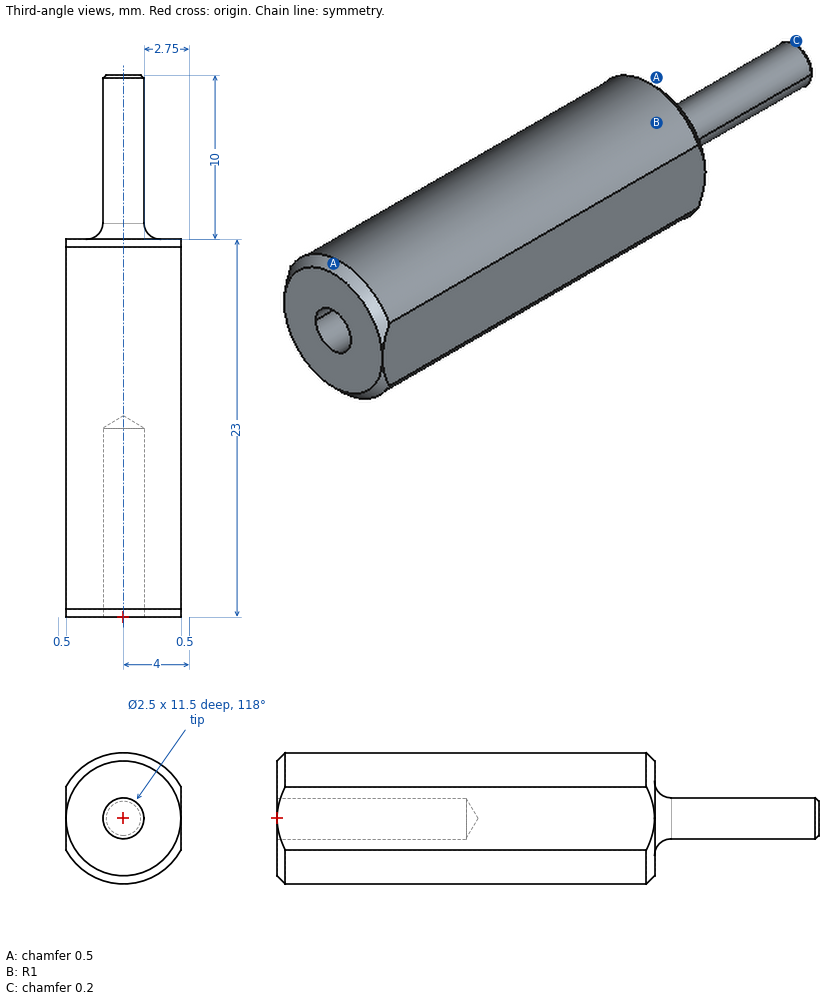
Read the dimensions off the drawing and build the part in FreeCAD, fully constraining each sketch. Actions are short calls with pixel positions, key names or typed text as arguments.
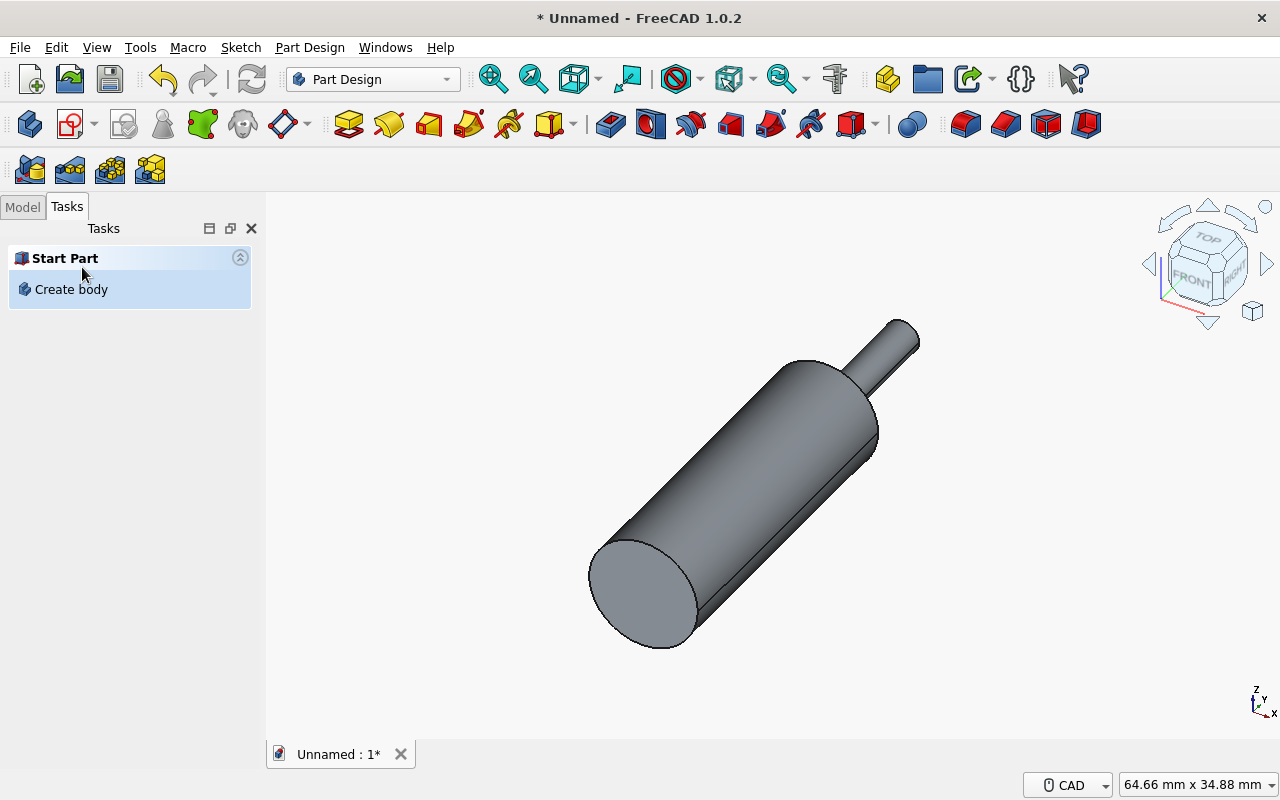
click(70, 124)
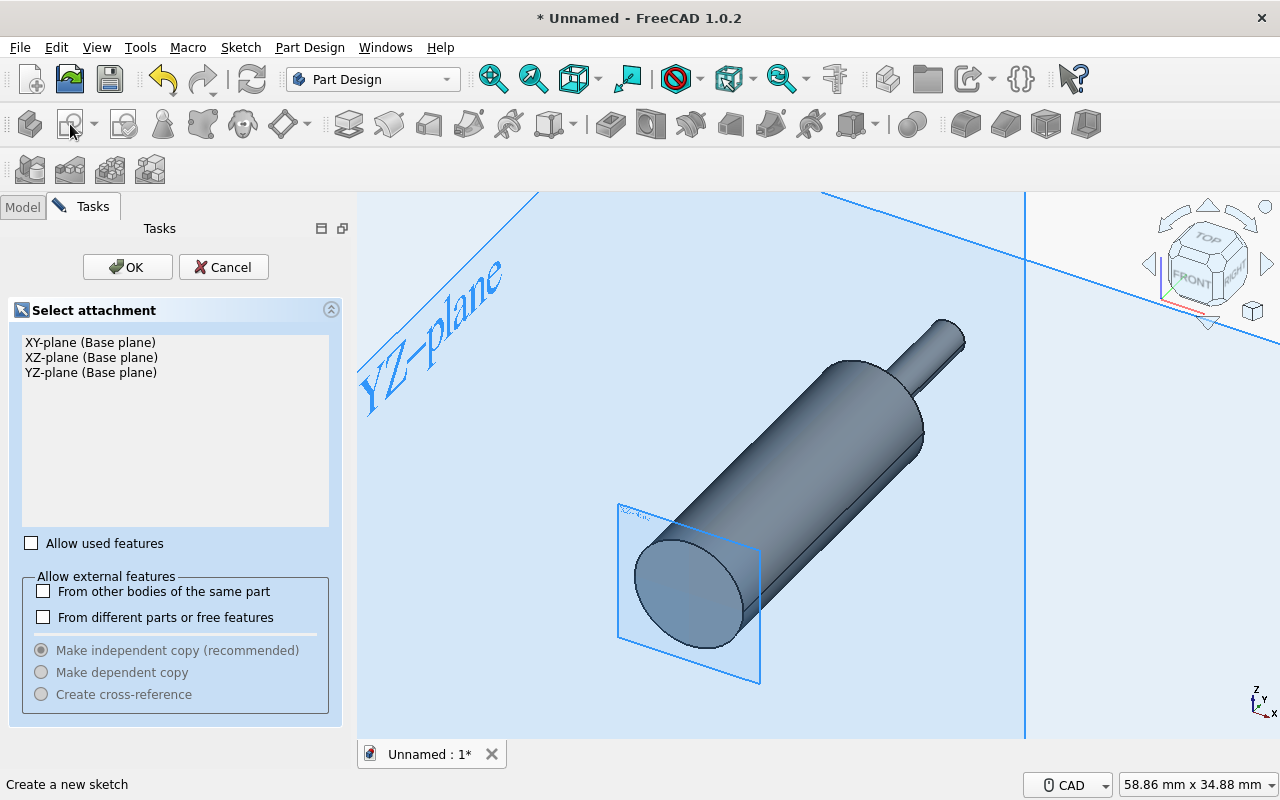
click(82, 358)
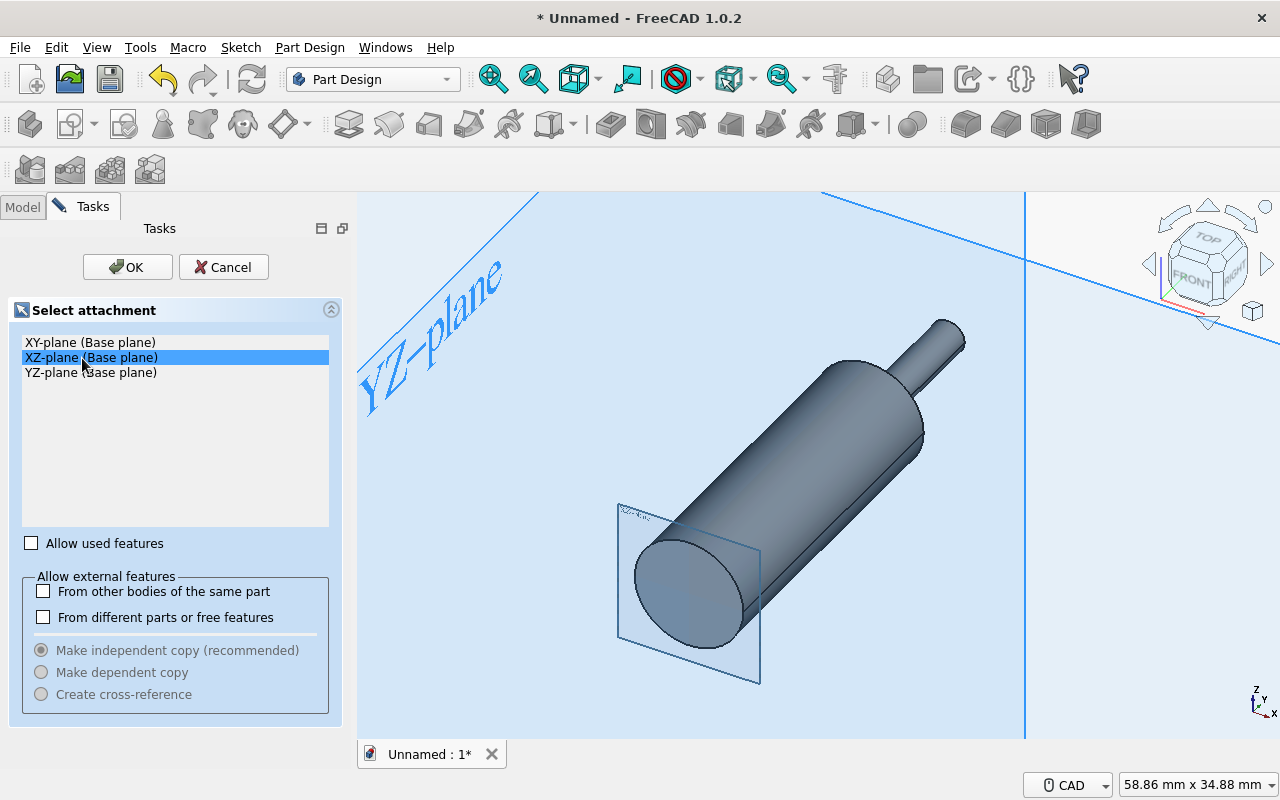
click(128, 267)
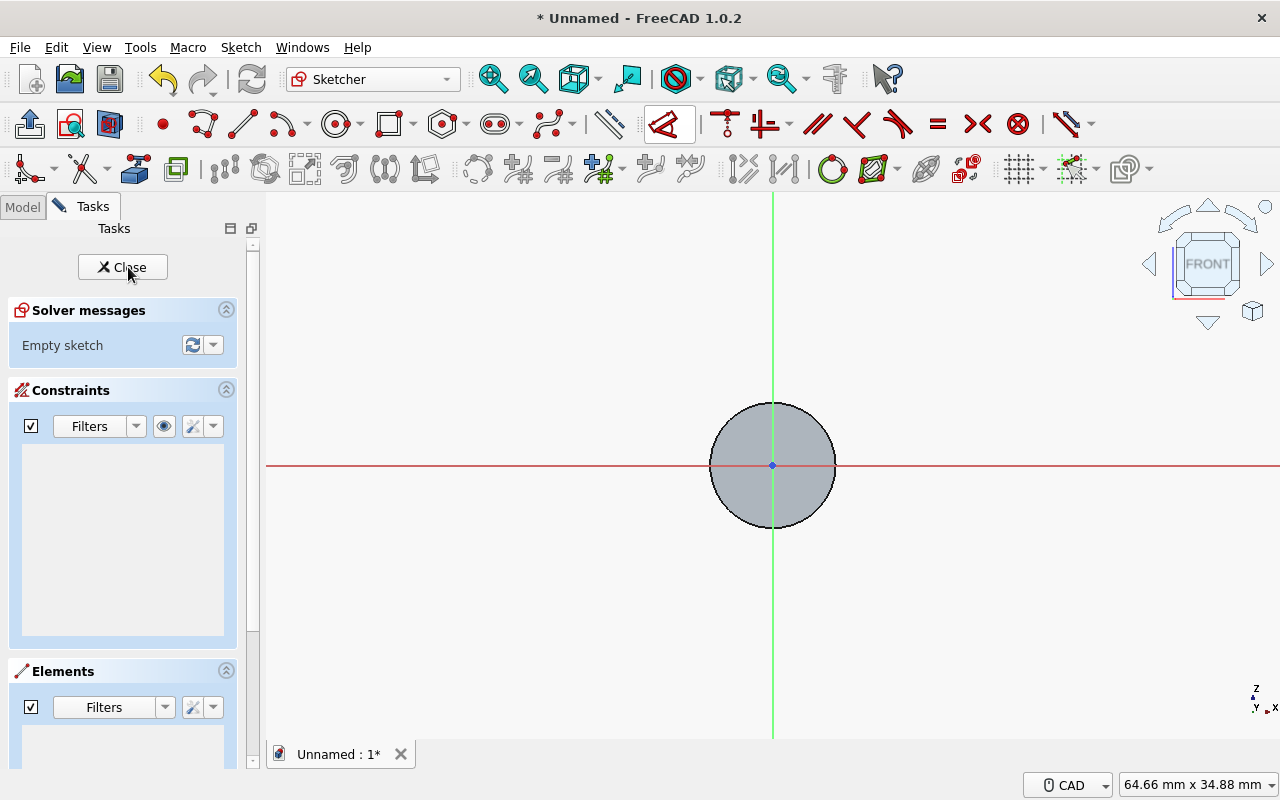
scroll(781, 466, up, 11)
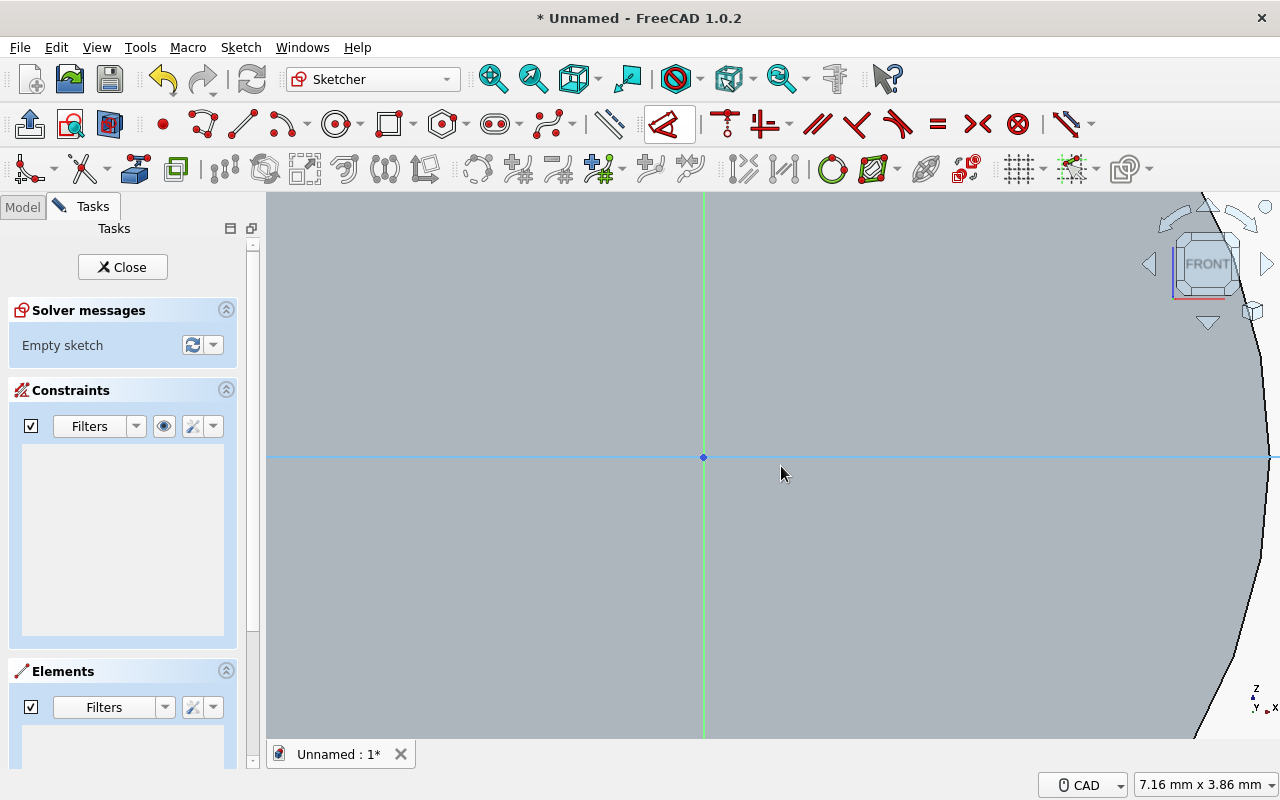
key(g)
key(c)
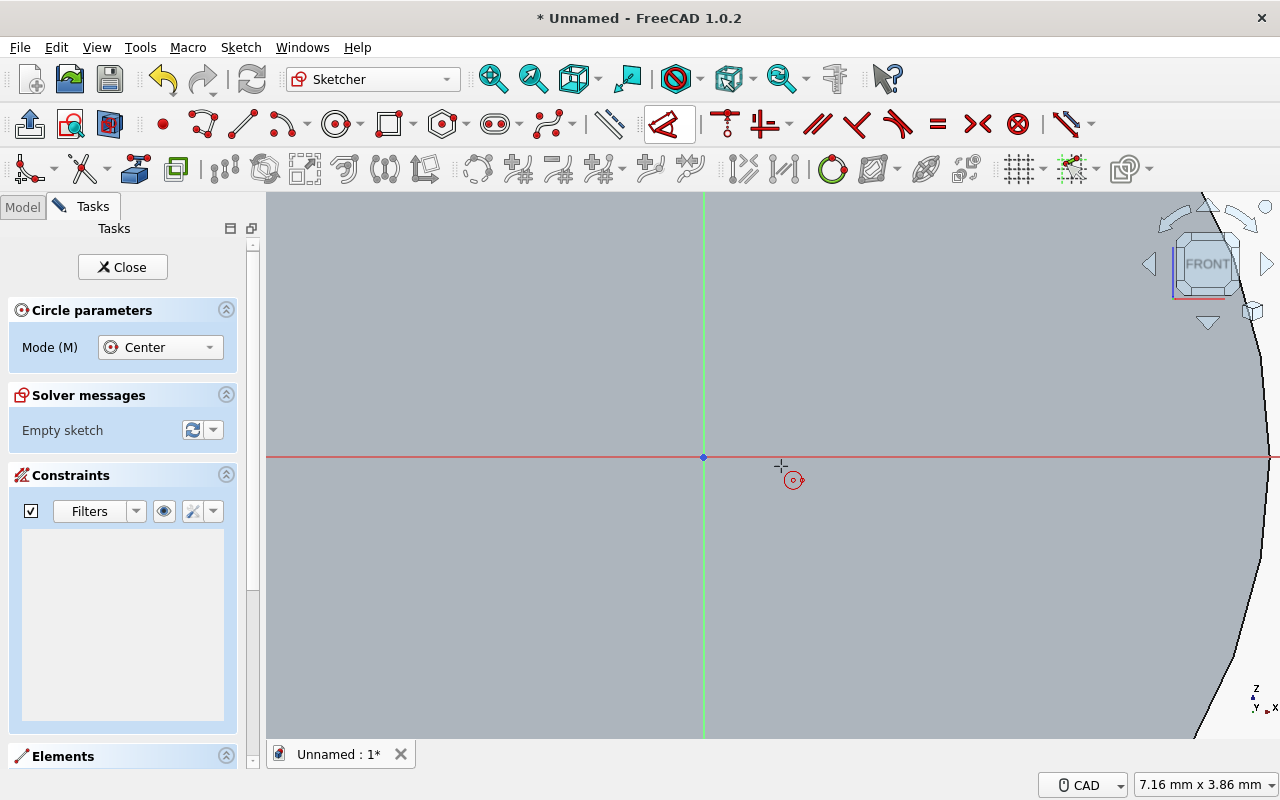
click(704, 457)
move(829, 332)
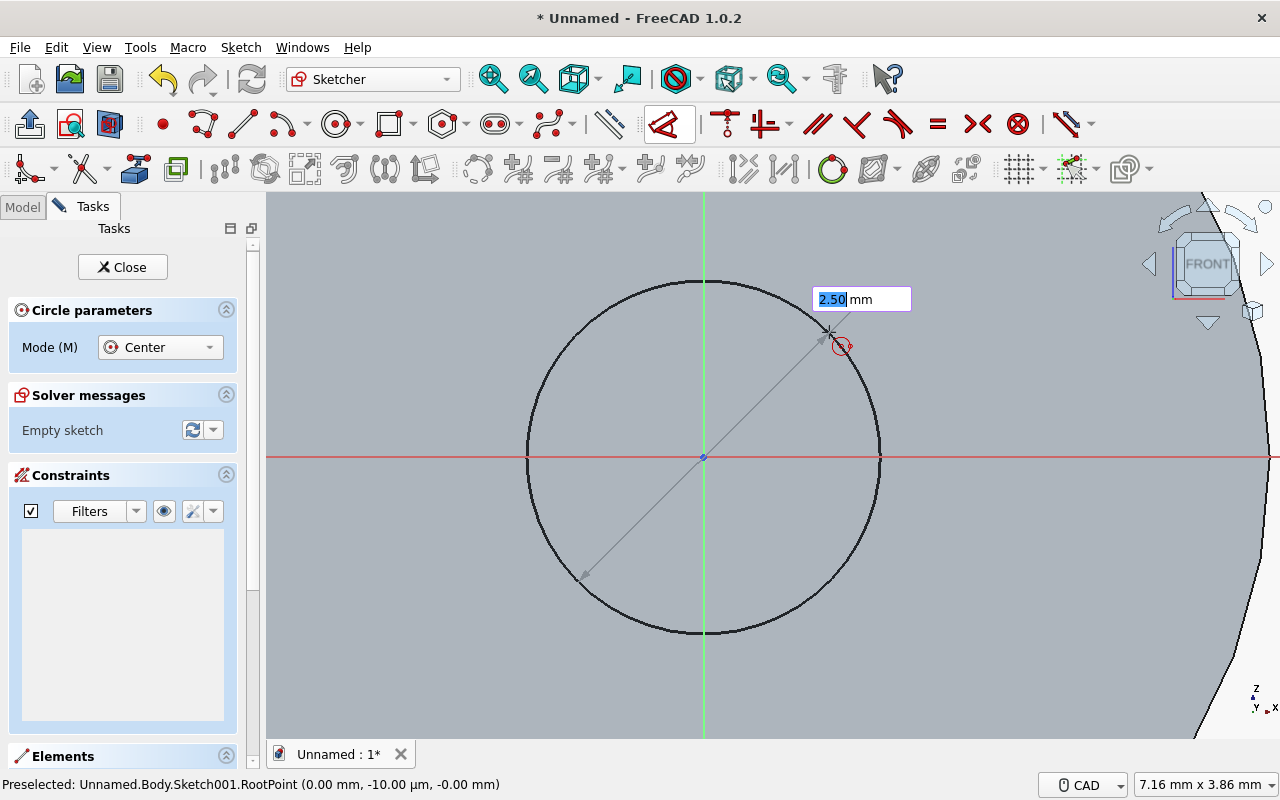
text(2.5)
key(Return)
key(Escape)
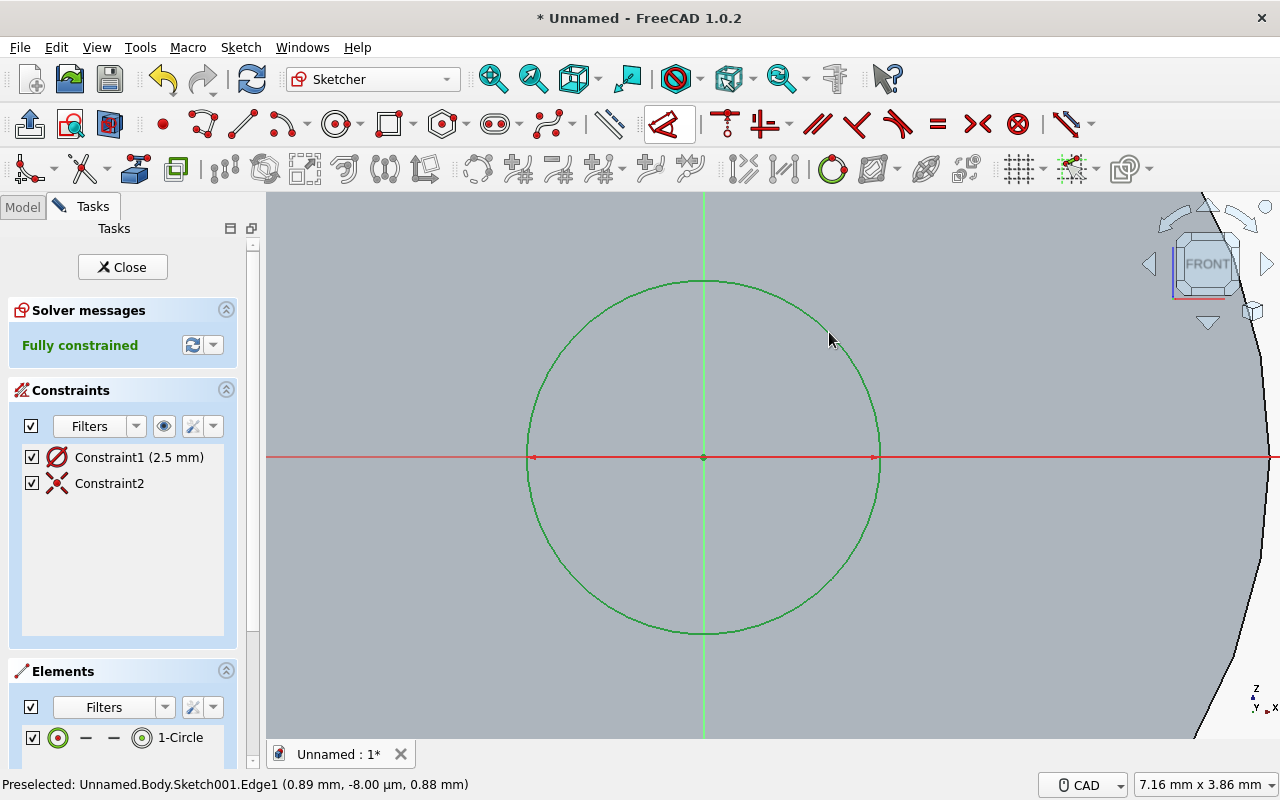
click(123, 267)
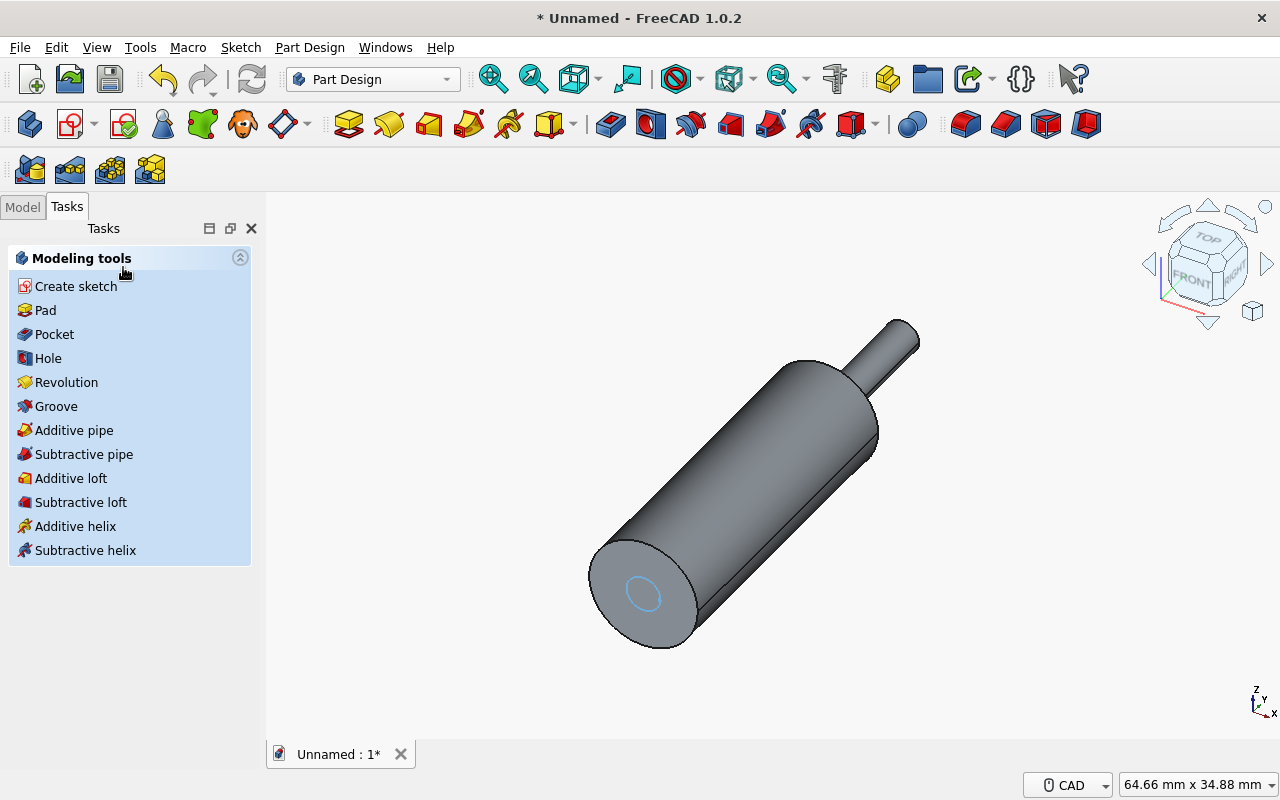
click(652, 124)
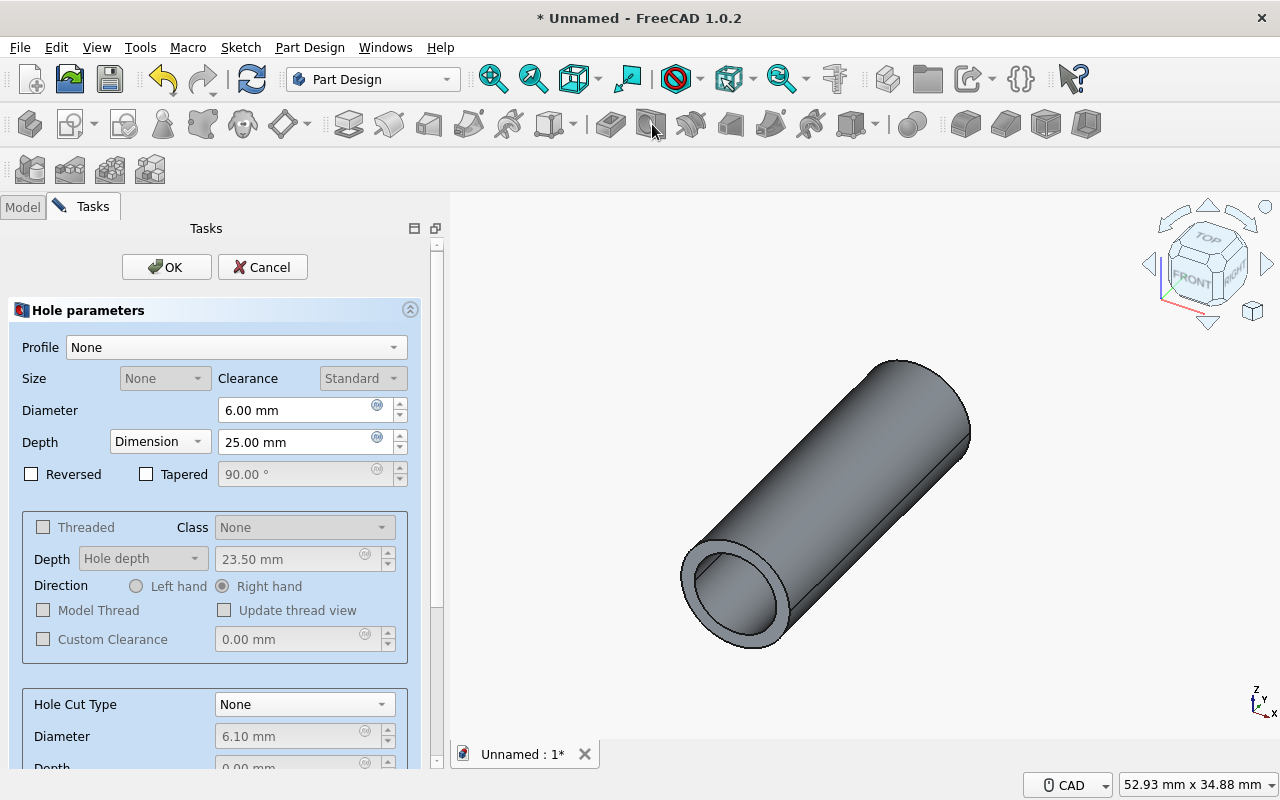
triple_click(305, 410)